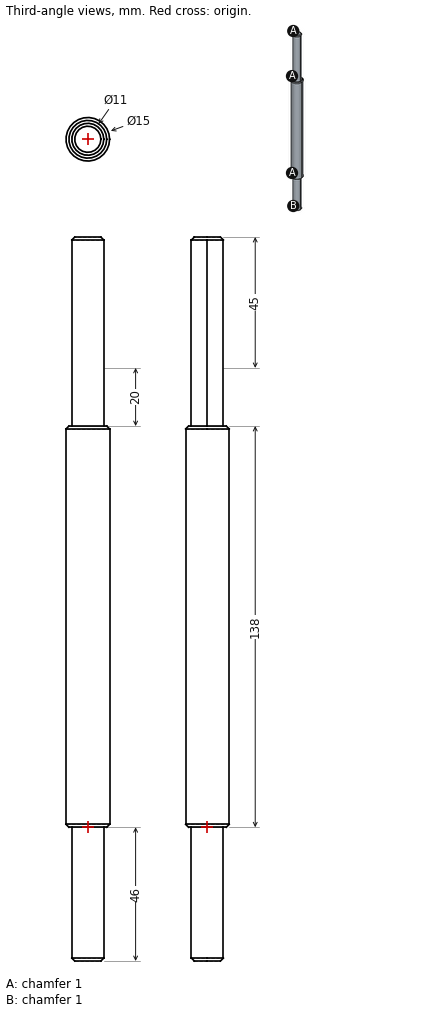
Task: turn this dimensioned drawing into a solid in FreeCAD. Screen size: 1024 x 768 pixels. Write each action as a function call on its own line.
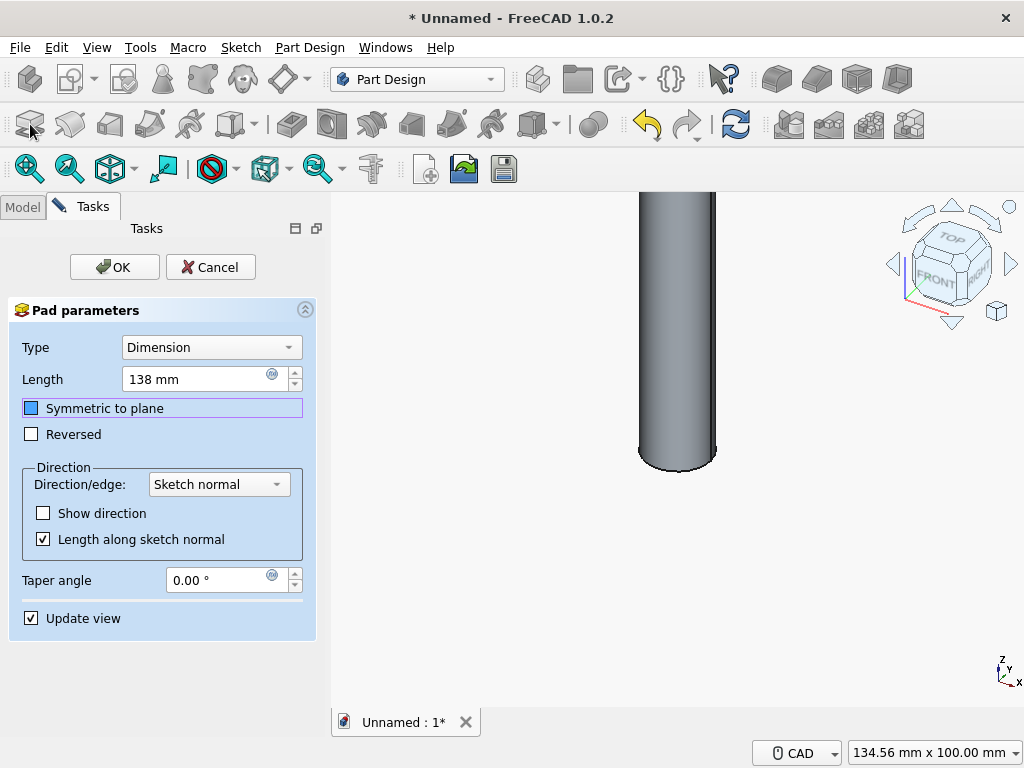
click(115, 267)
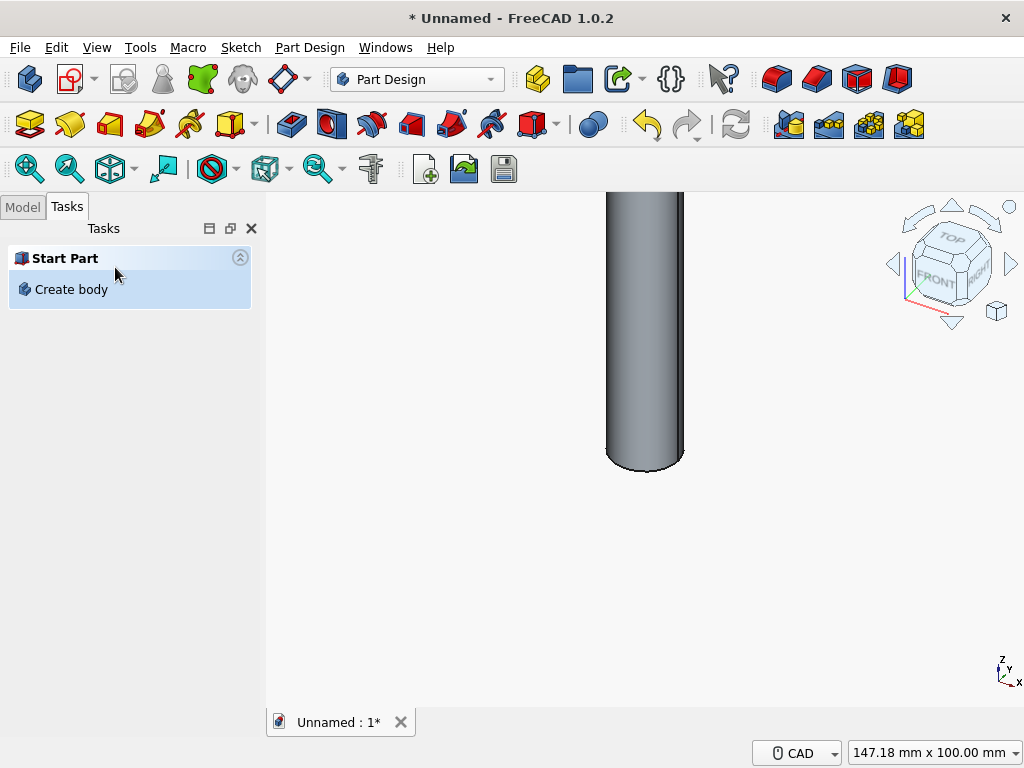
click(30, 170)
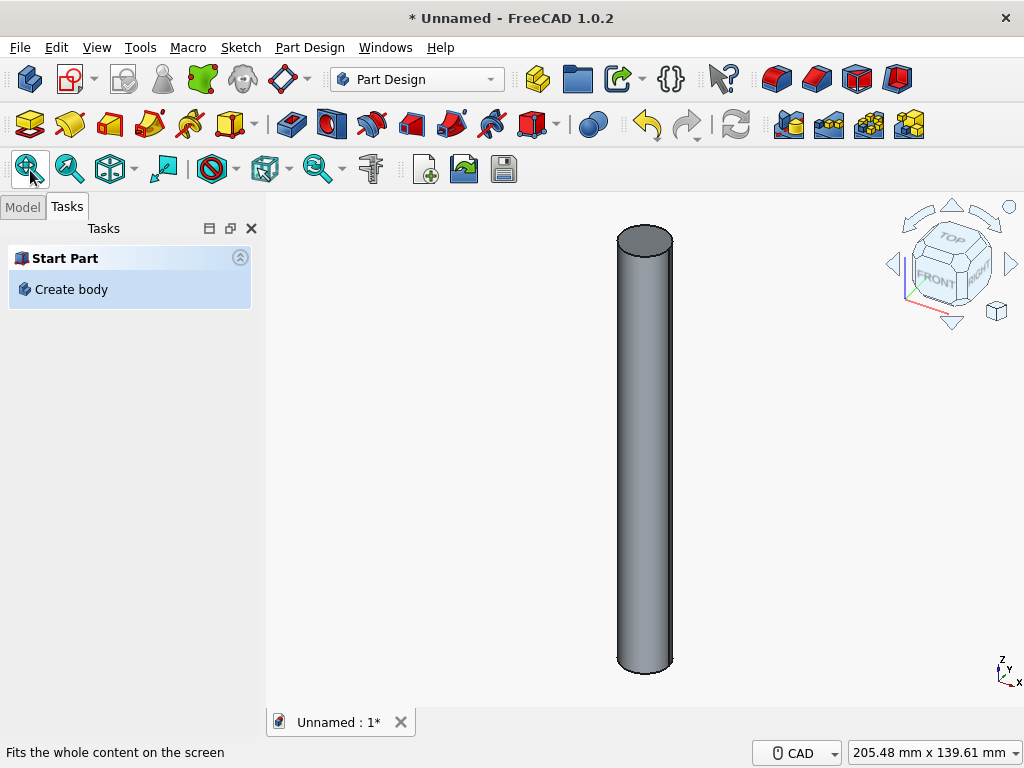
click(645, 240)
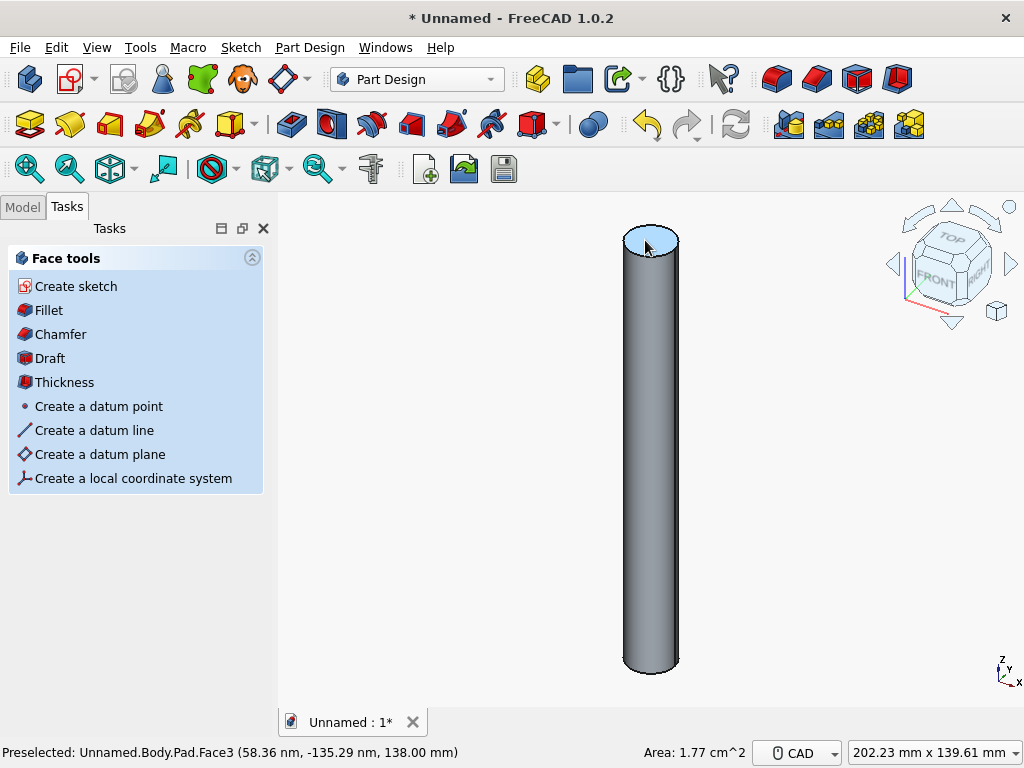
click(70, 80)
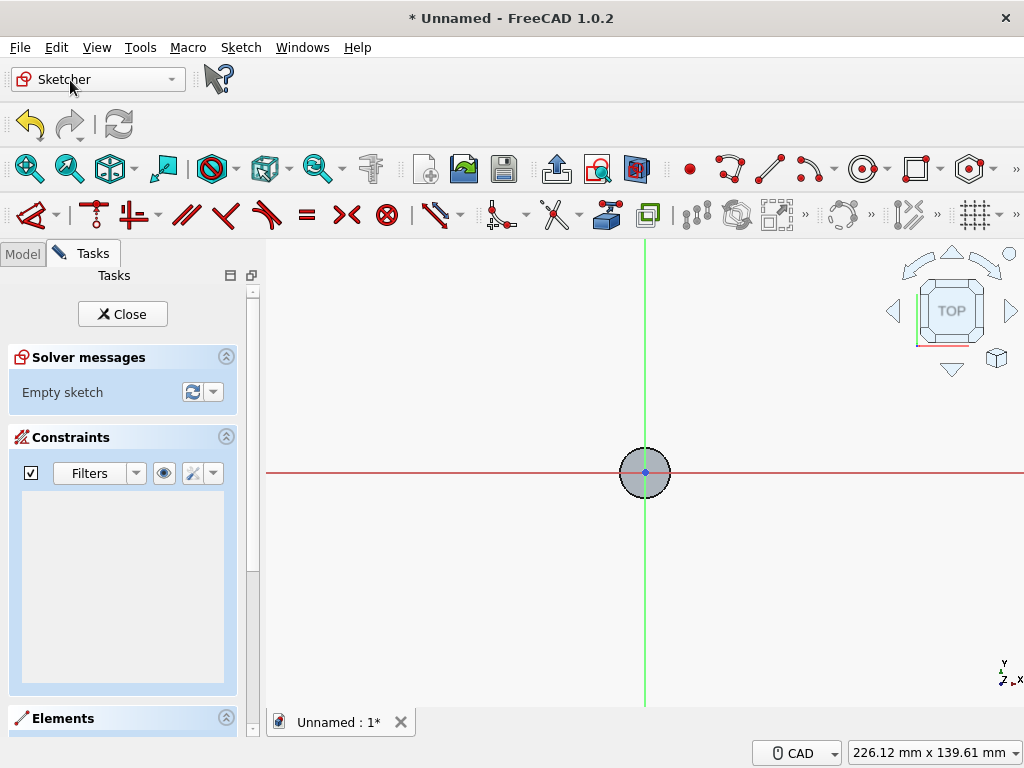
scroll(656, 473, up, 10)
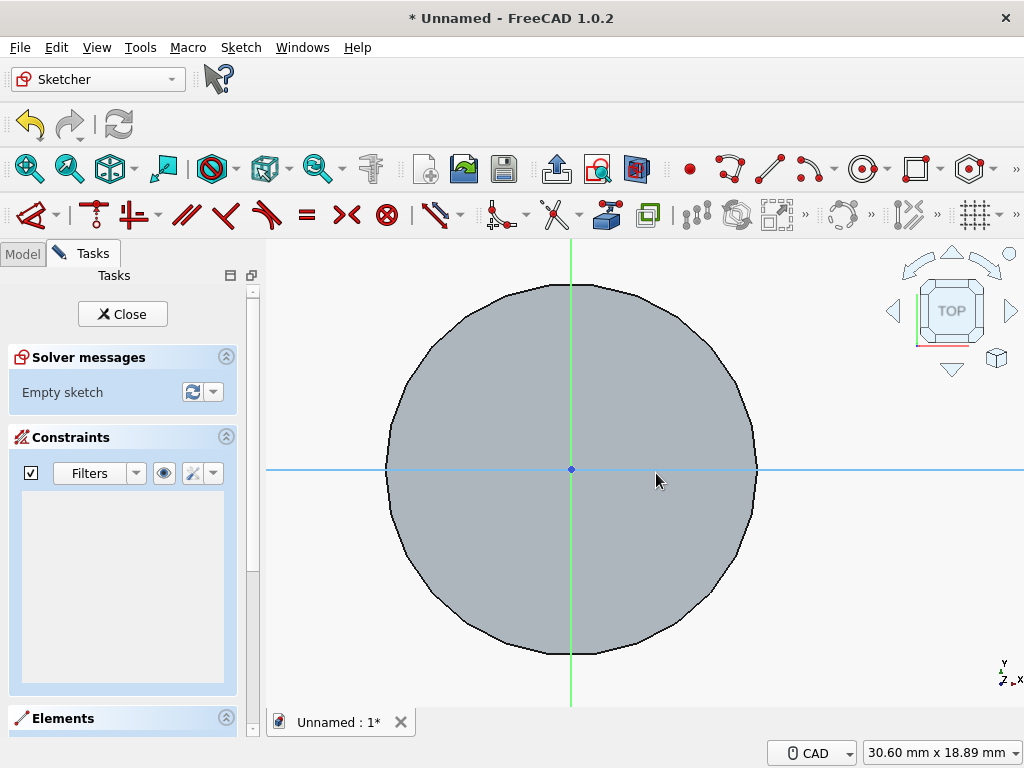
click(864, 170)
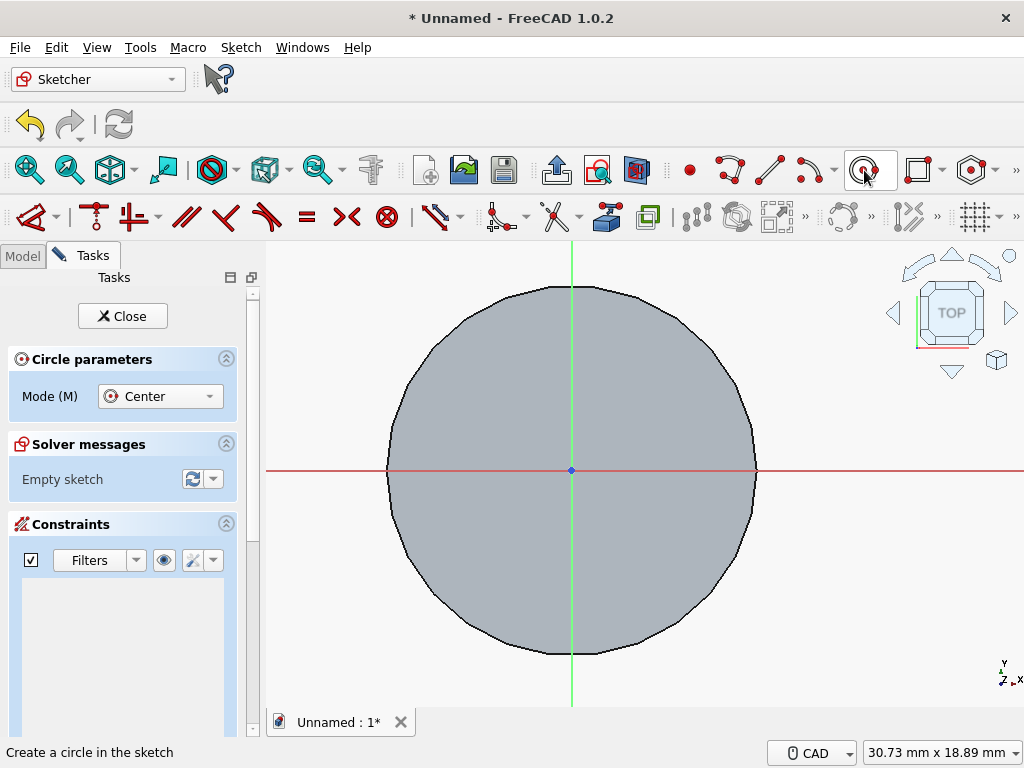
click(572, 471)
click(668, 375)
key(Escape)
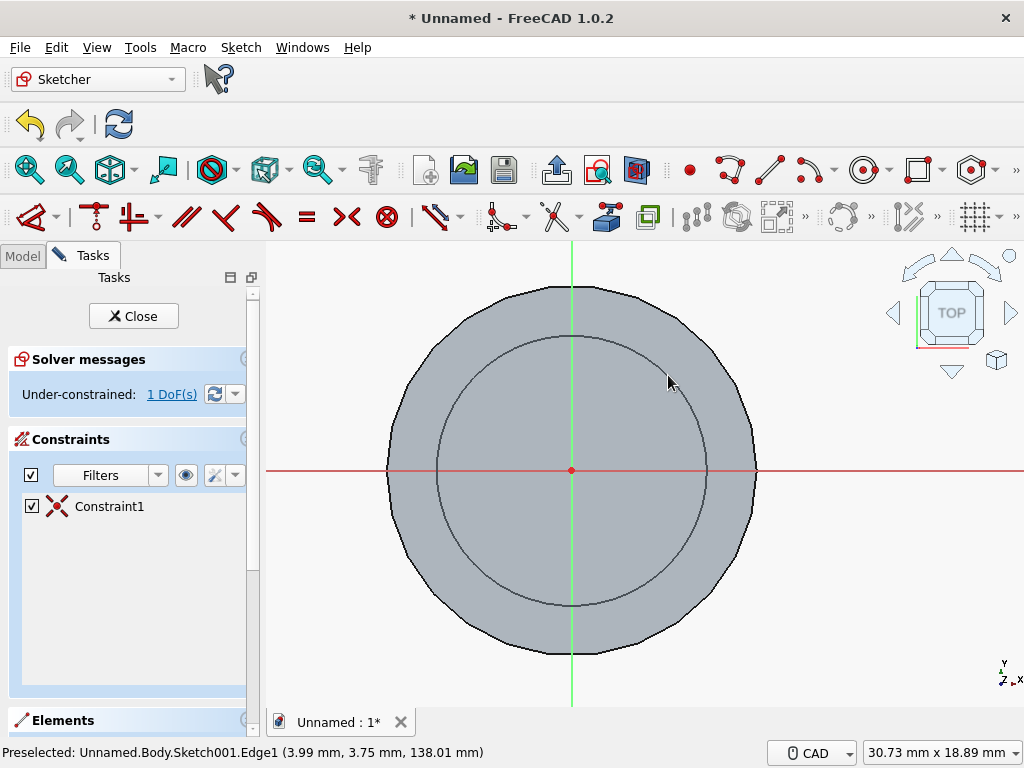
click(32, 218)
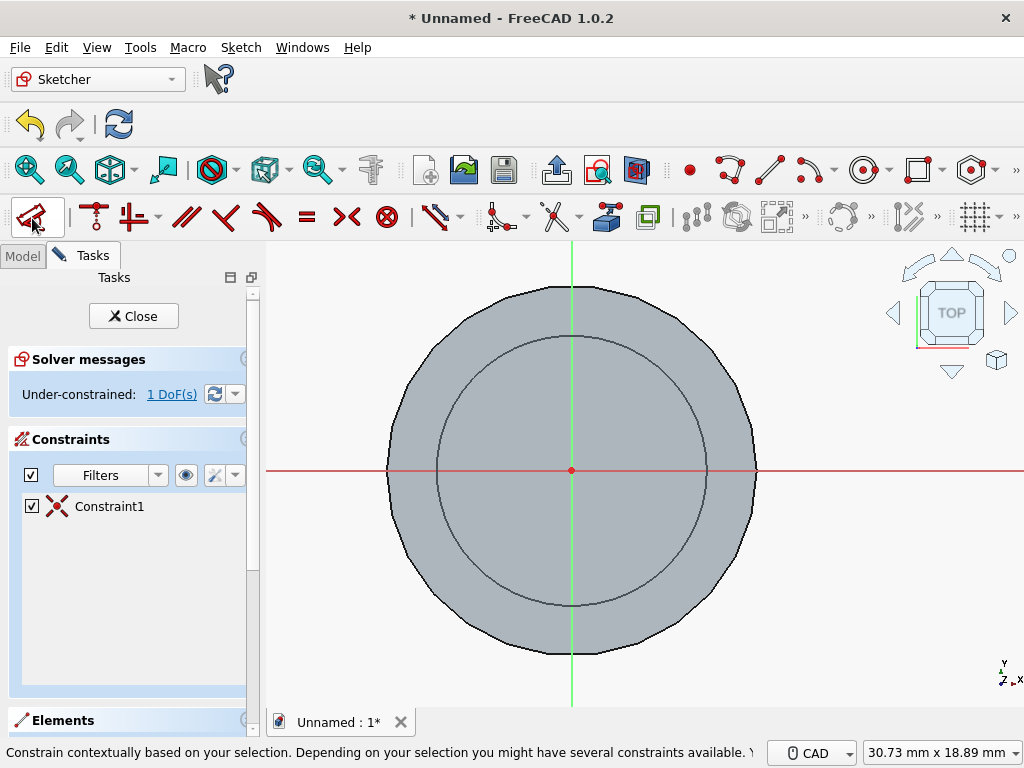
click(667, 375)
click(690, 352)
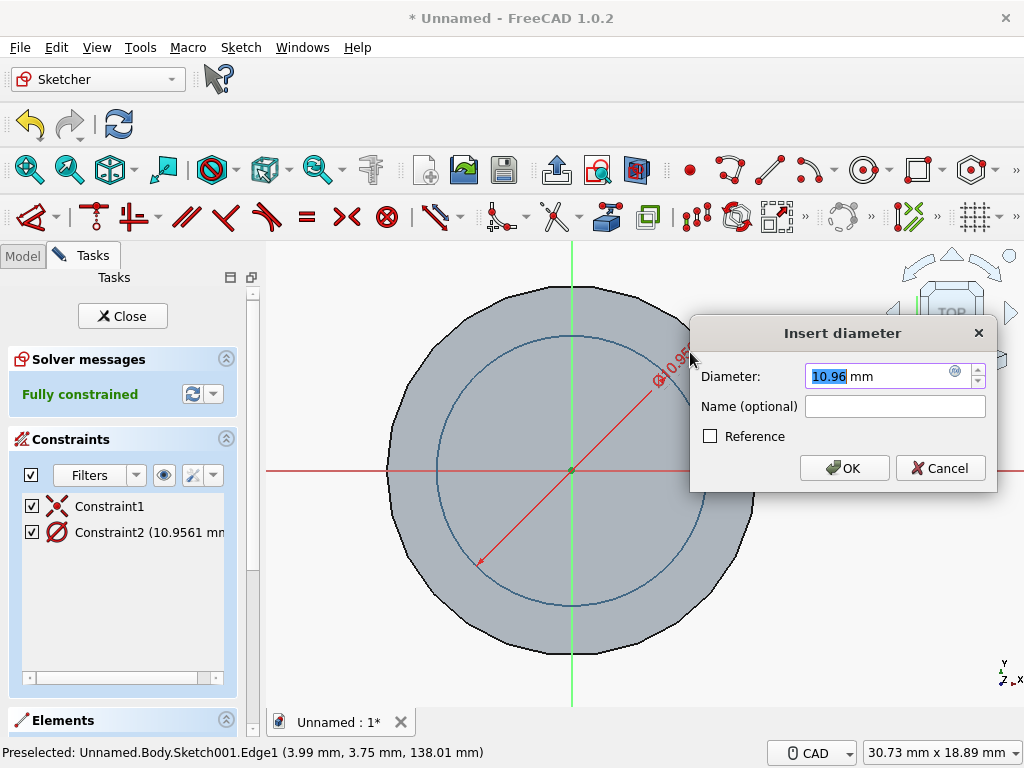
text(11)
key(Return)
key(Escape)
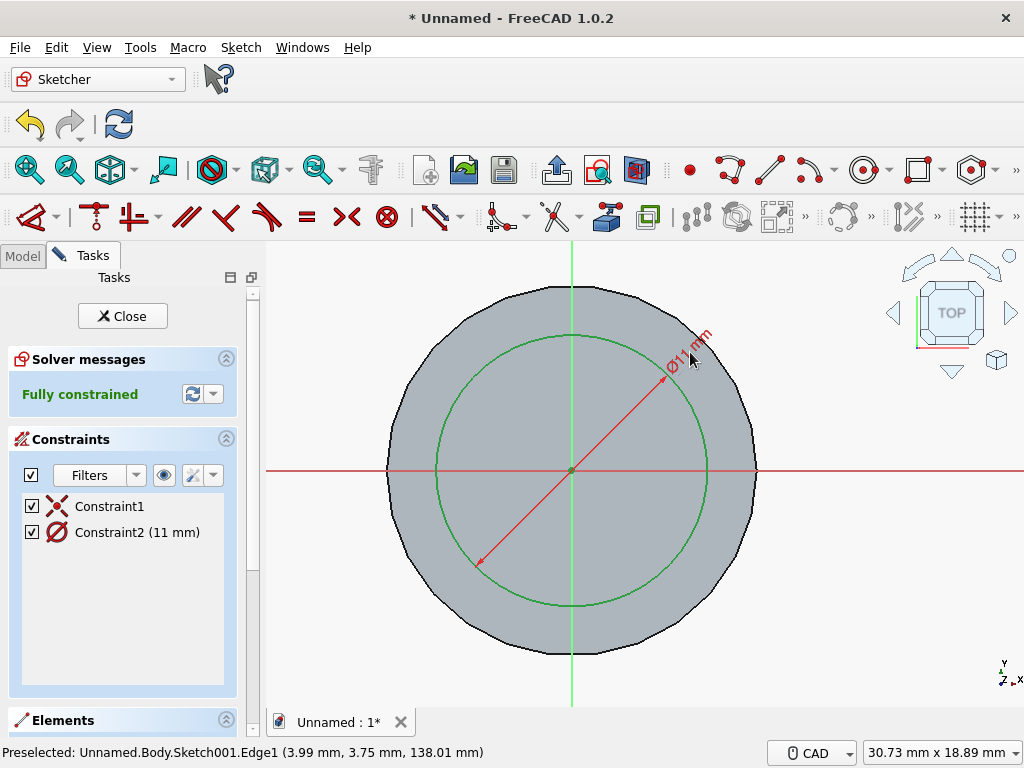
click(123, 316)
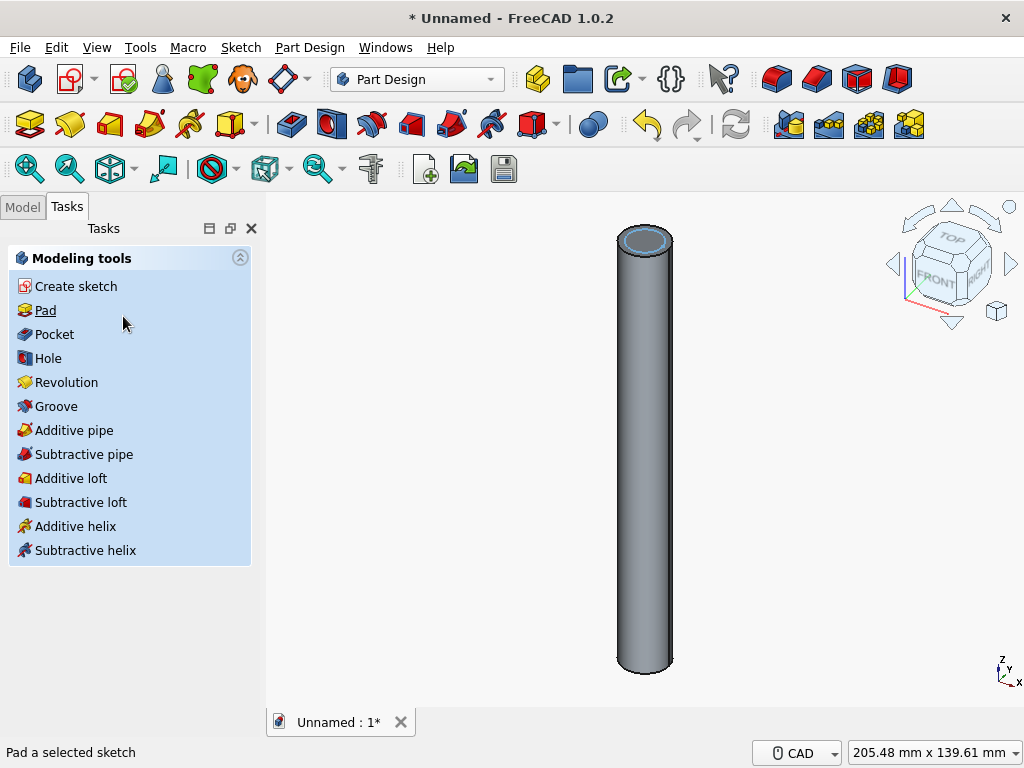
click(30, 124)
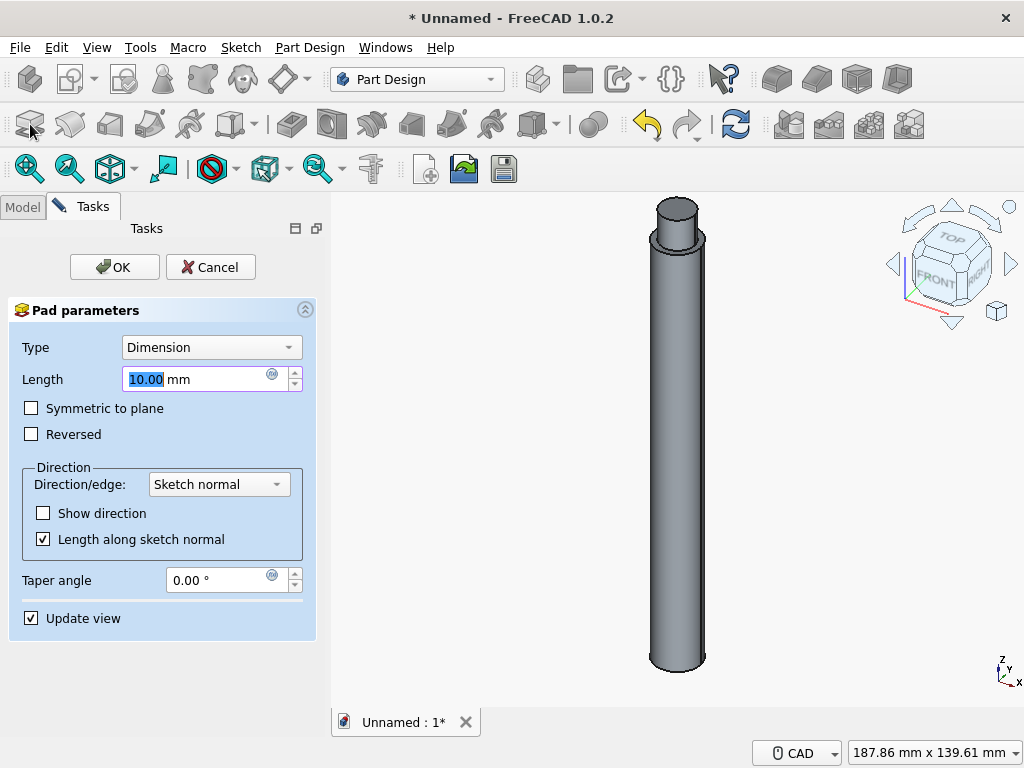
text(20)
key(Tab)